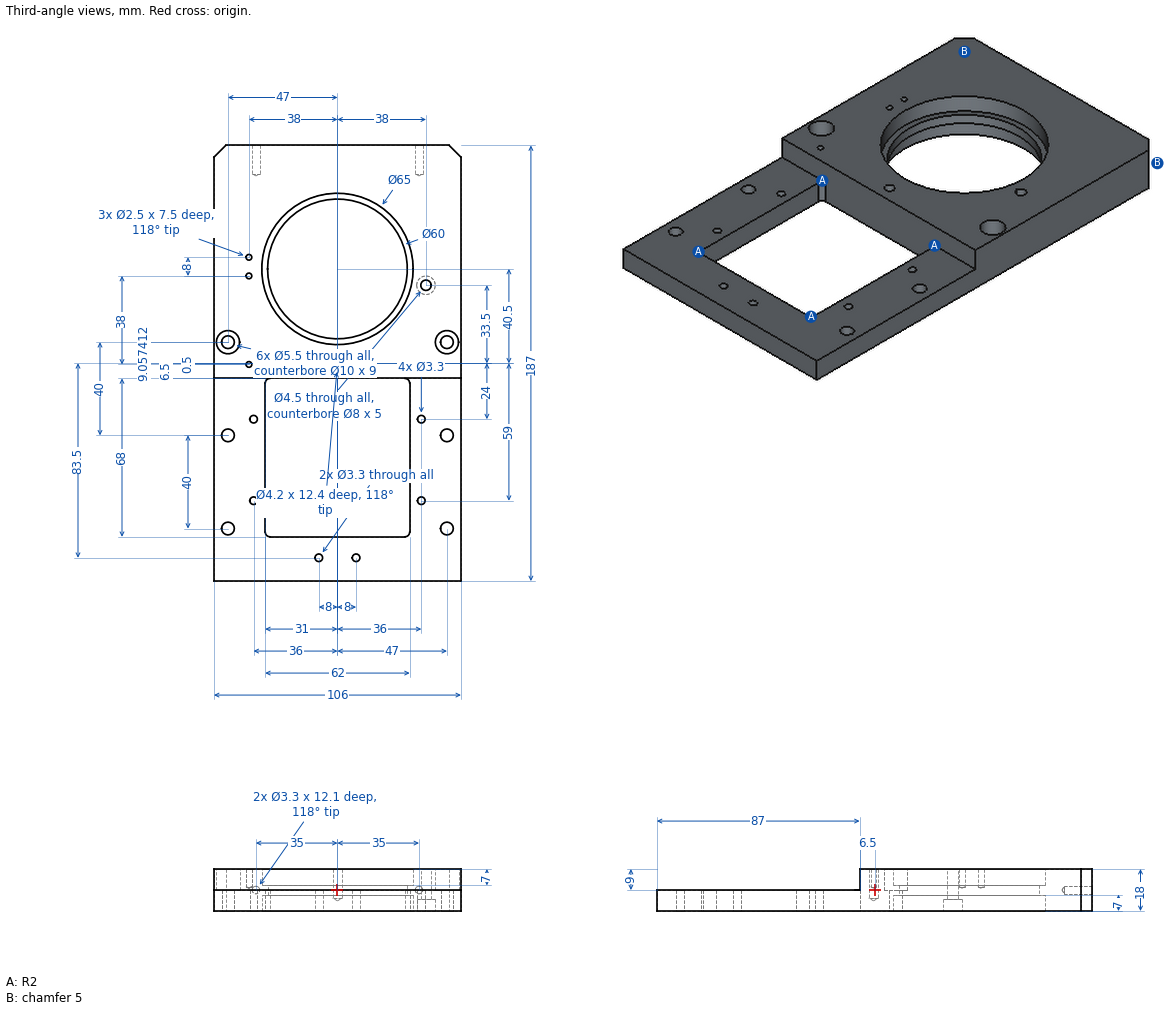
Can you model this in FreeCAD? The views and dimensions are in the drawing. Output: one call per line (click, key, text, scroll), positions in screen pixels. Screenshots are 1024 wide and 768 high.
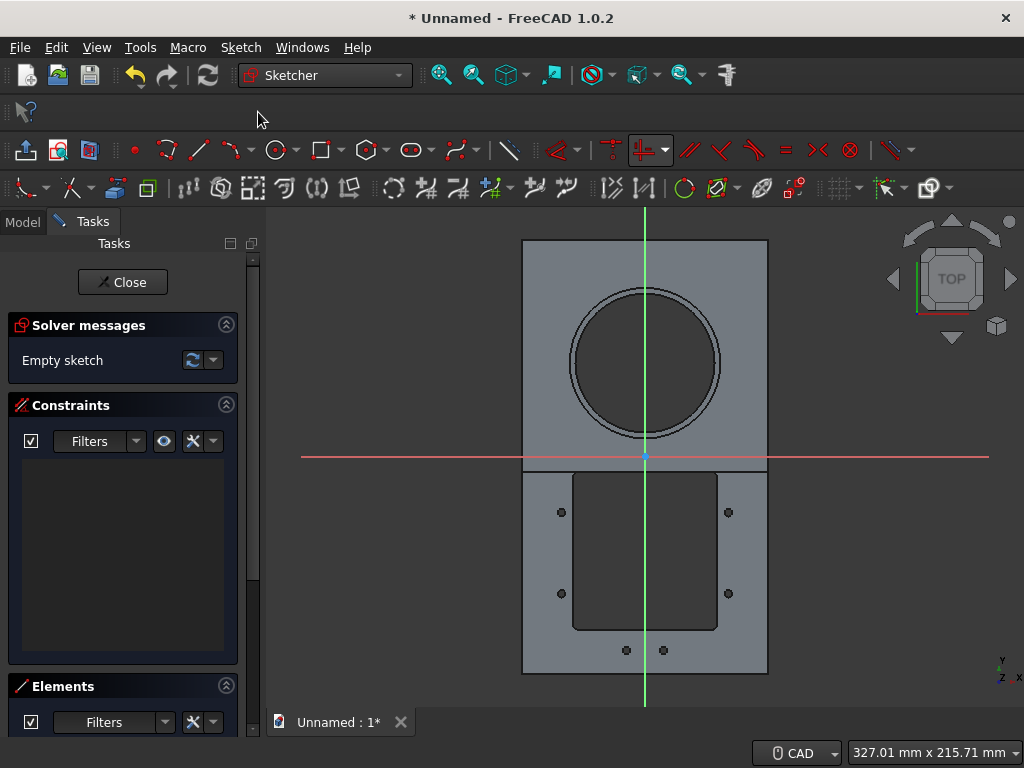
scroll(613, 374, up, 5)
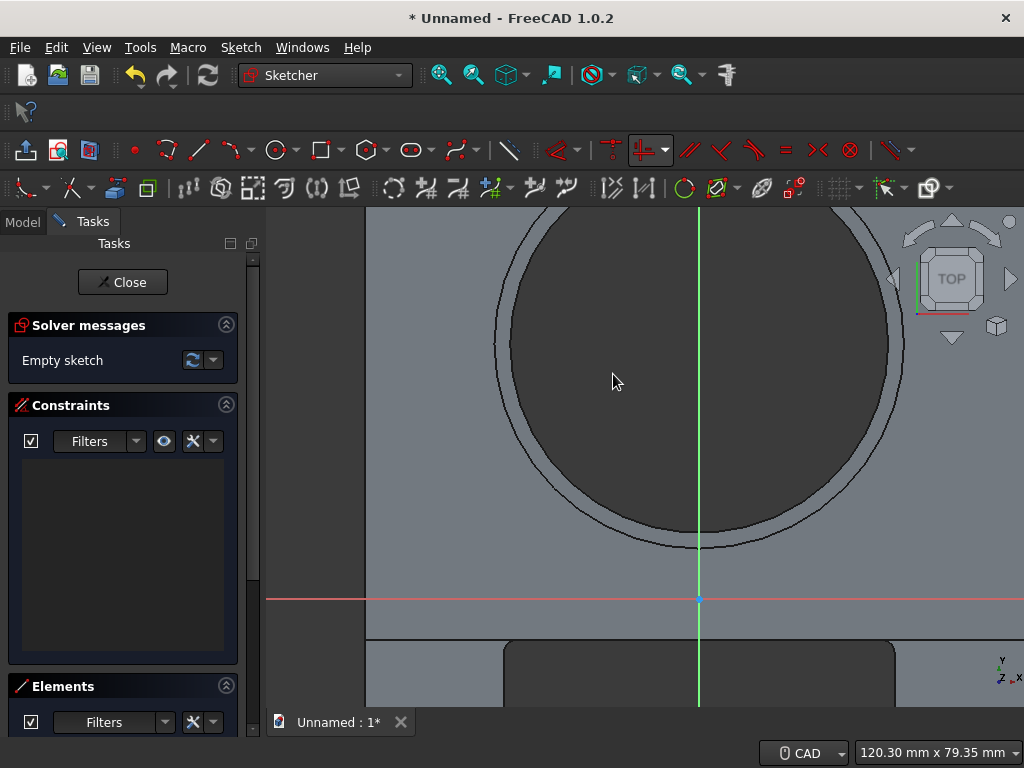
click(276, 150)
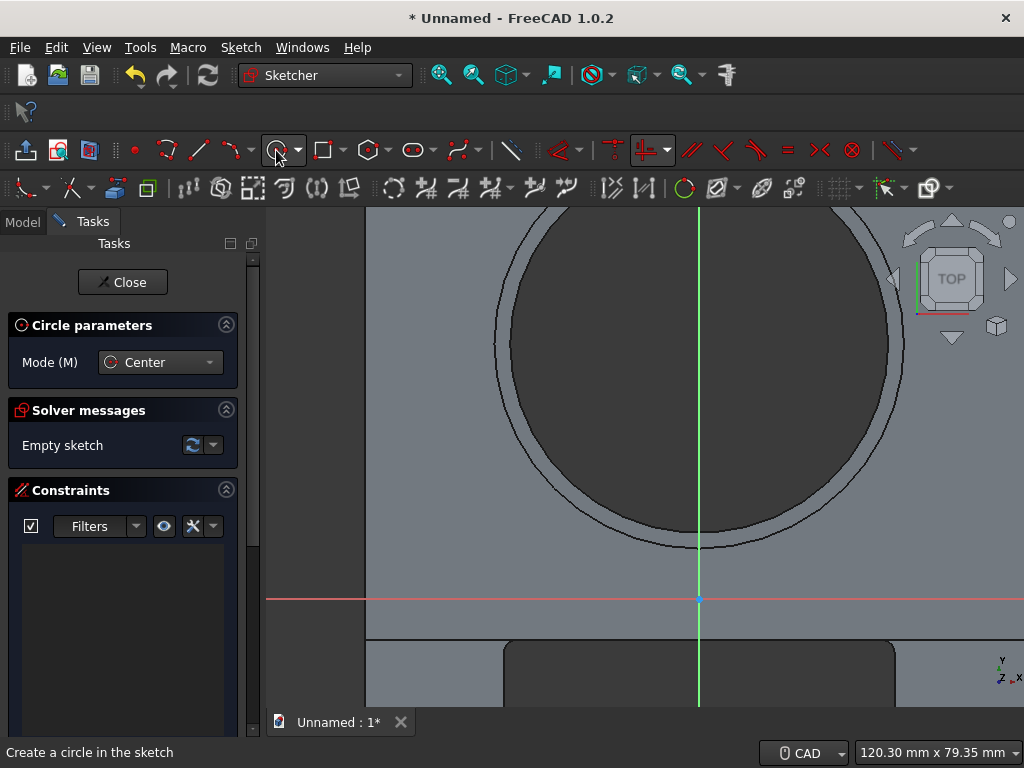
scroll(460, 312, up, 6)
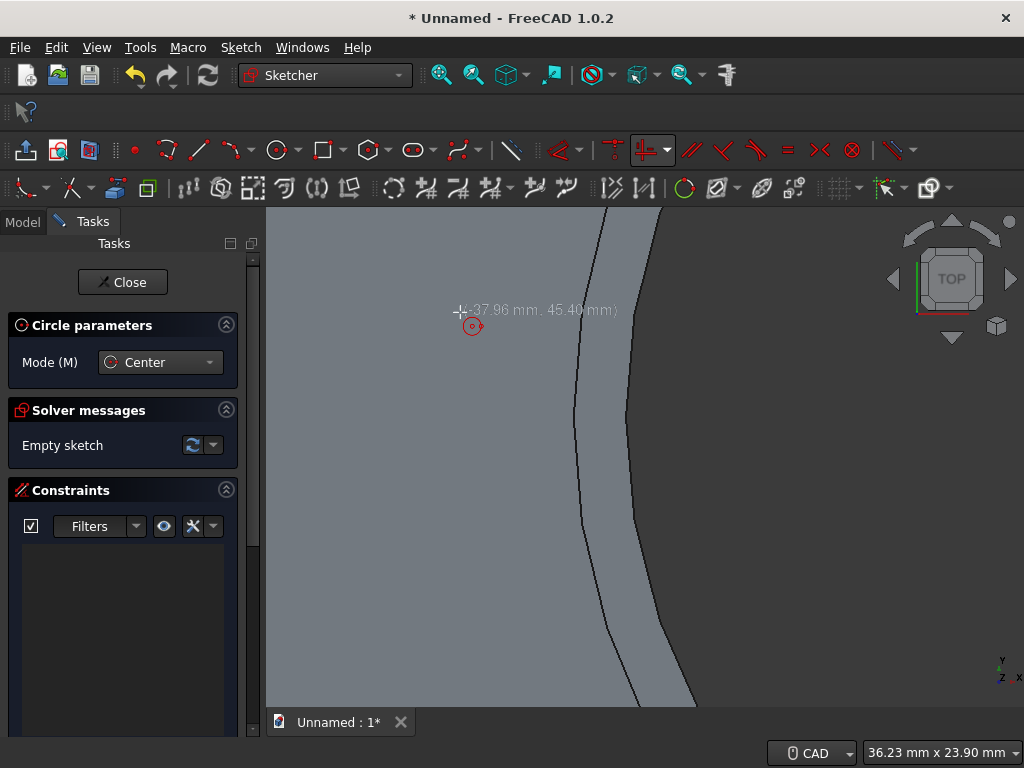
click(459, 313)
click(477, 294)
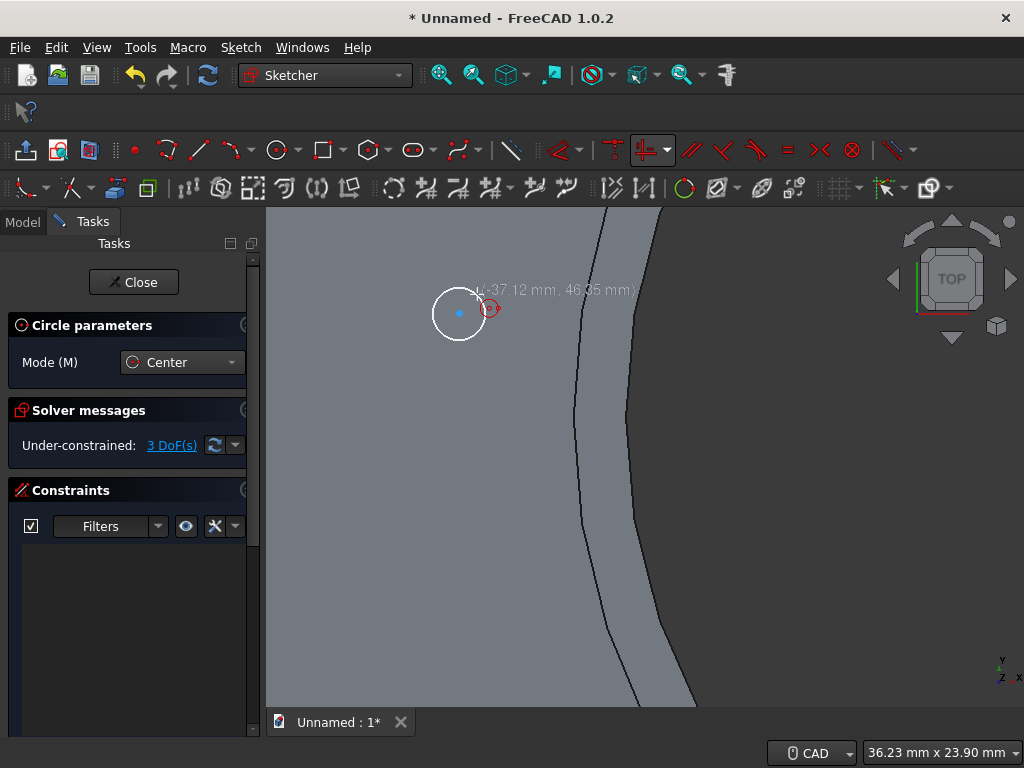
click(459, 480)
click(477, 462)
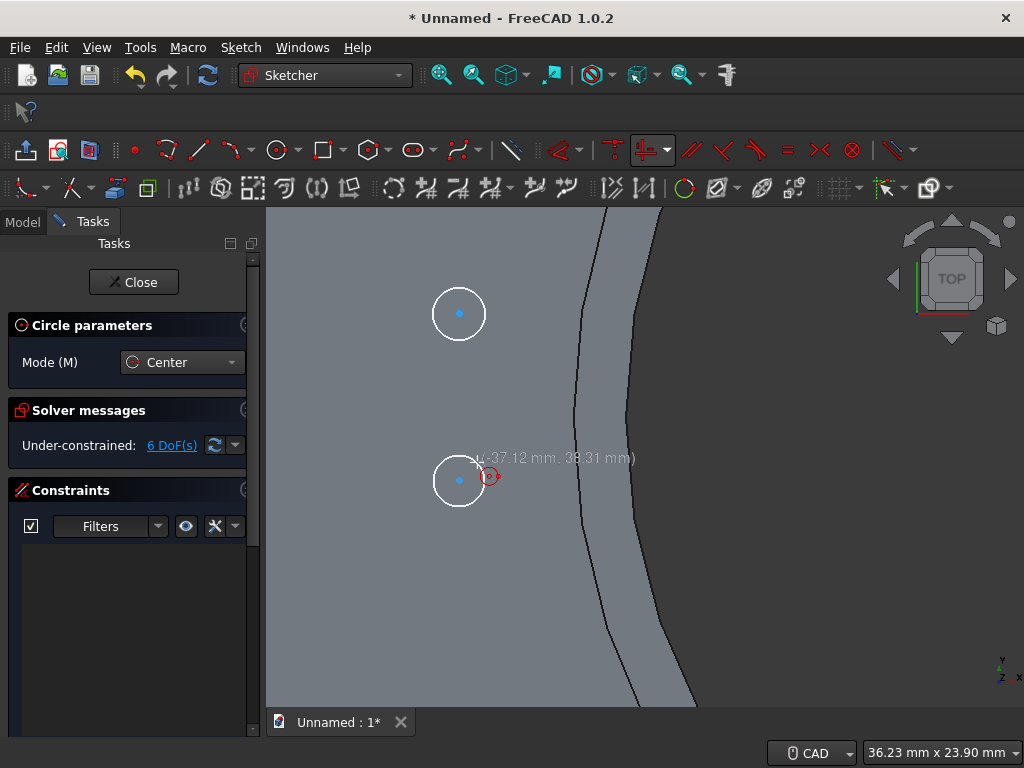
scroll(462, 312, down, 6)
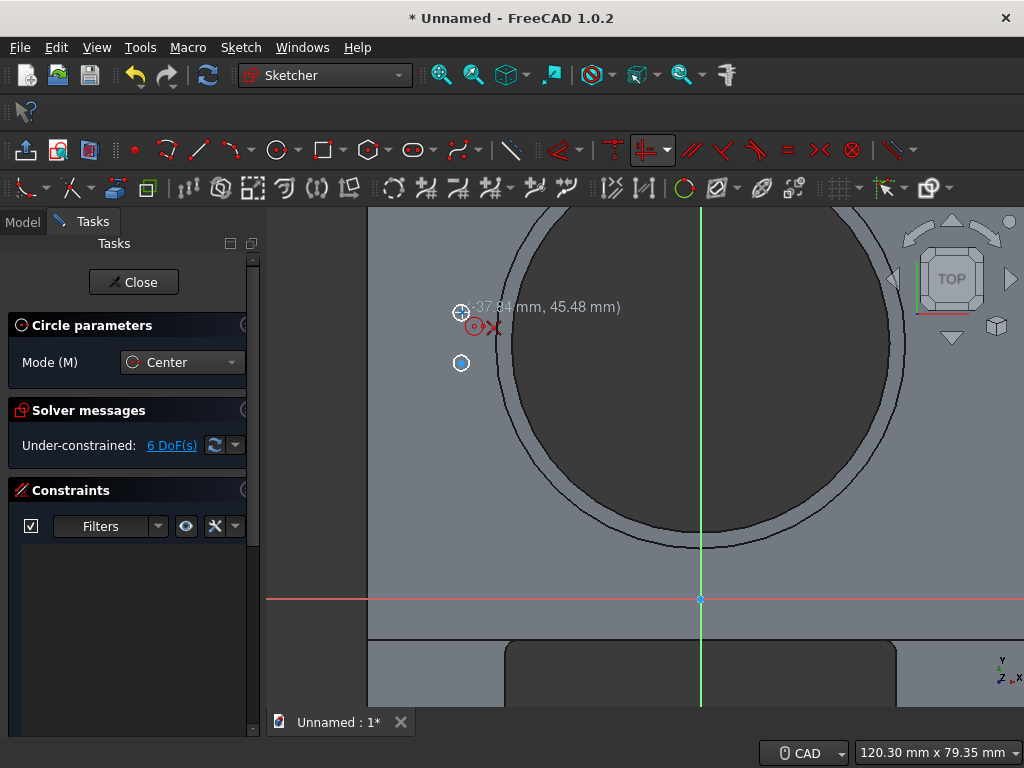
scroll(461, 602, up, 9)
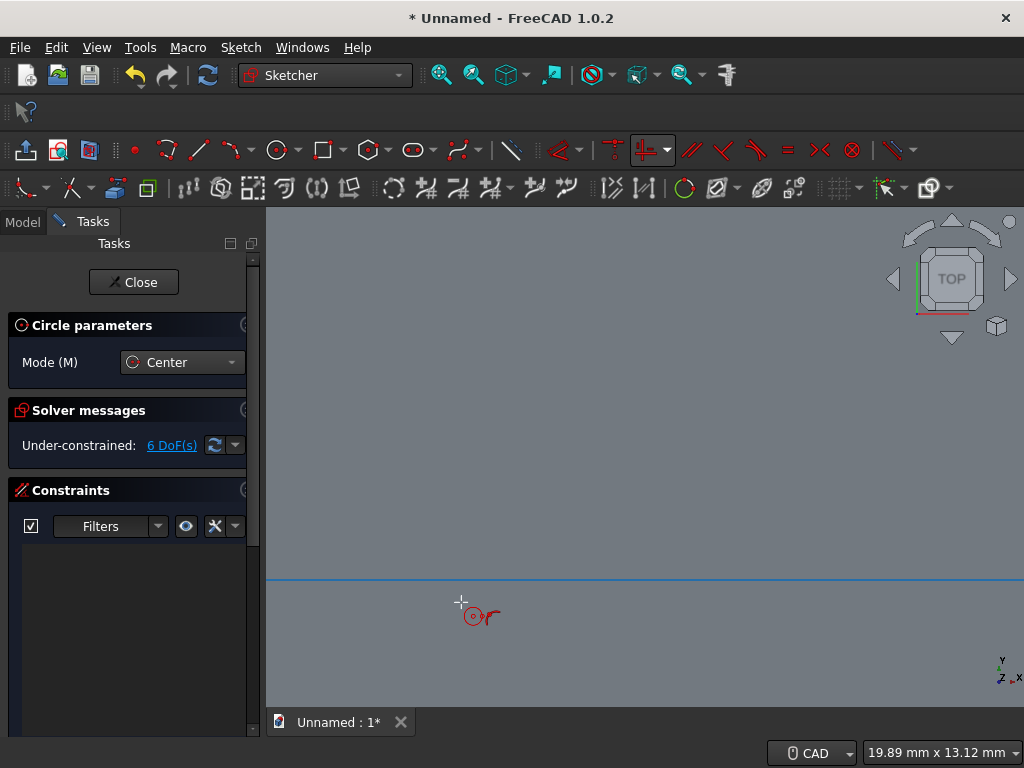
click(461, 599)
click(494, 565)
key(Escape)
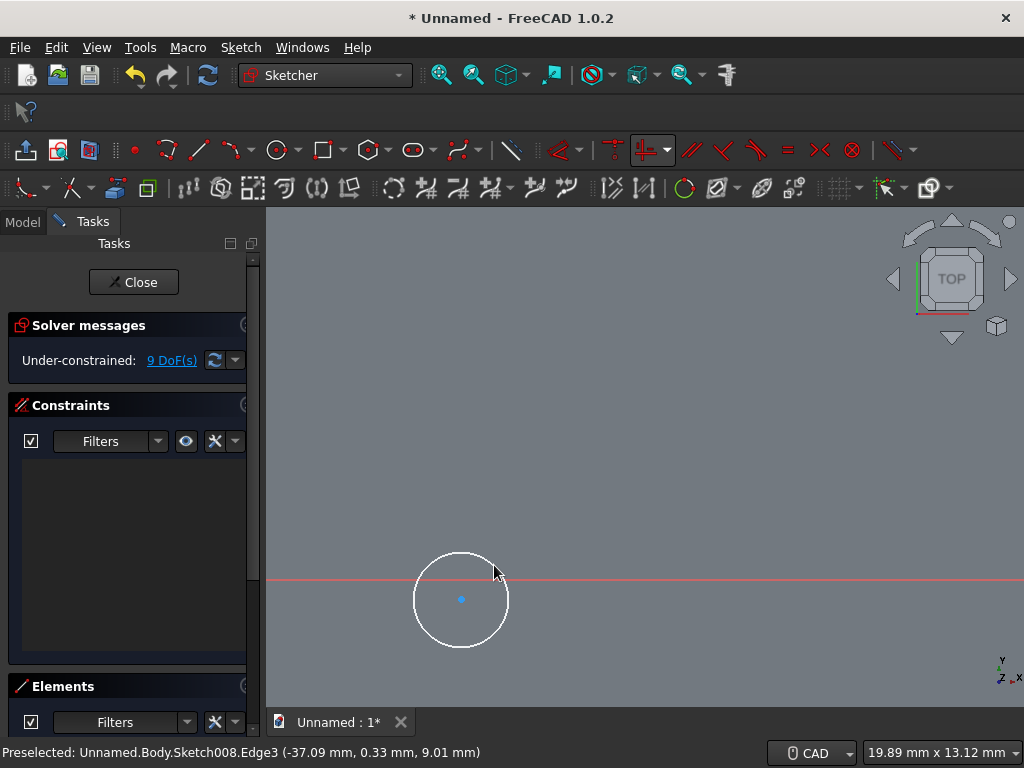
scroll(461, 602, down, 9)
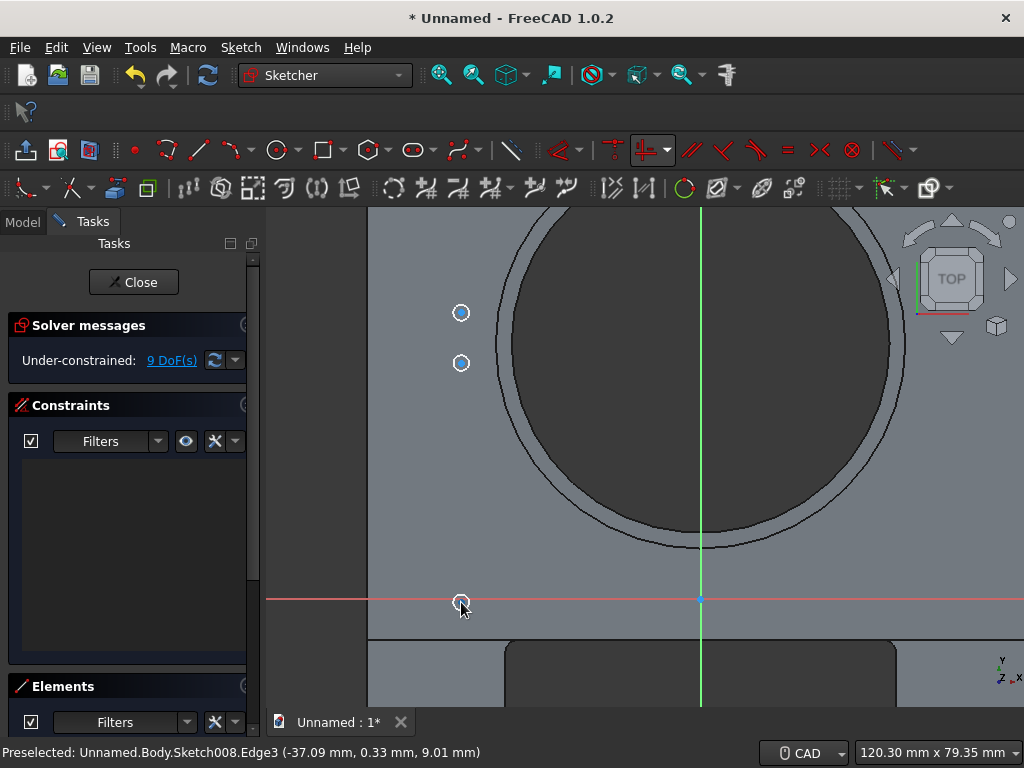
scroll(467, 307, up, 3)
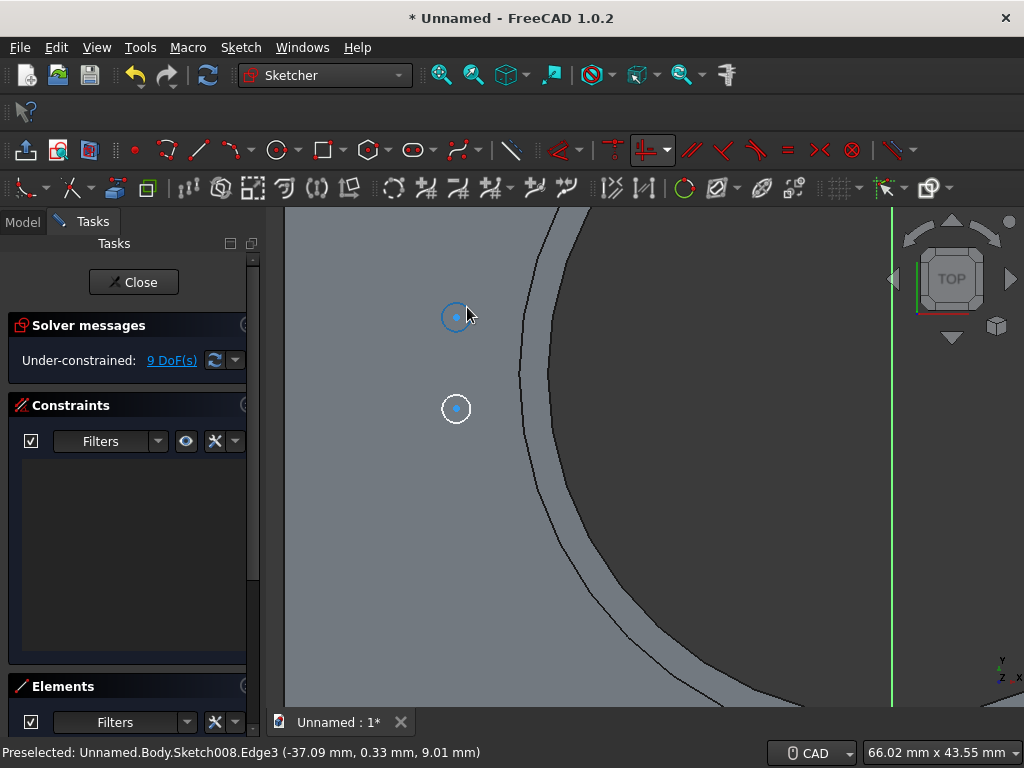
click(466, 307)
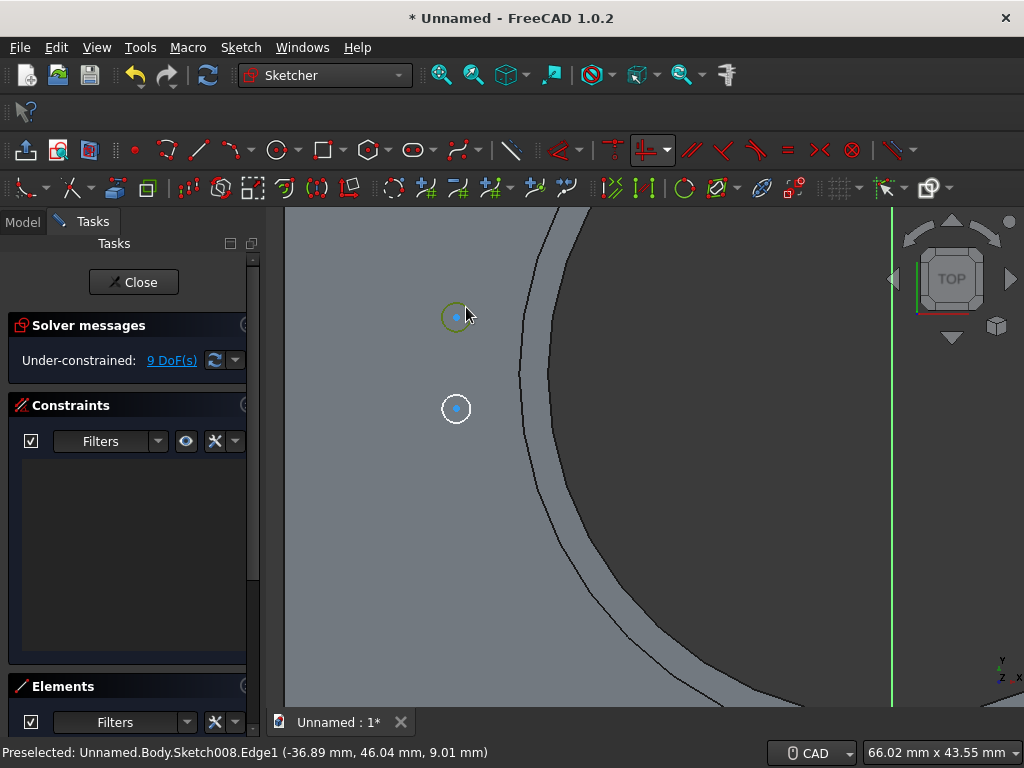
click(466, 399)